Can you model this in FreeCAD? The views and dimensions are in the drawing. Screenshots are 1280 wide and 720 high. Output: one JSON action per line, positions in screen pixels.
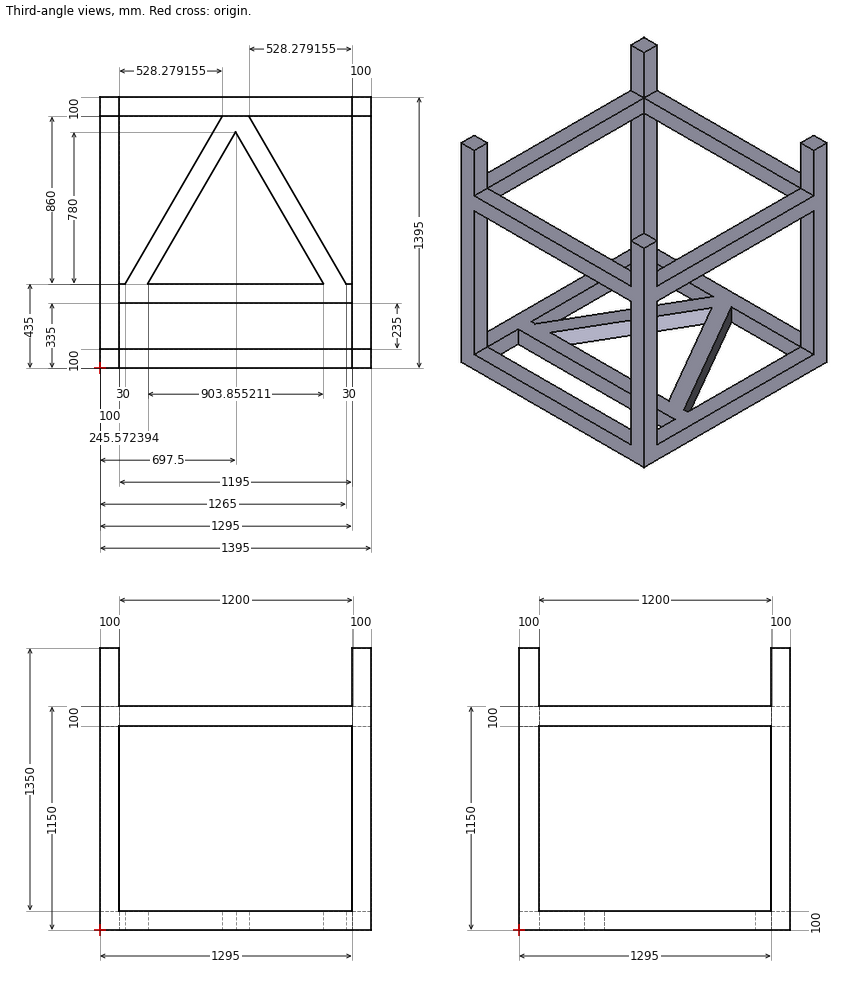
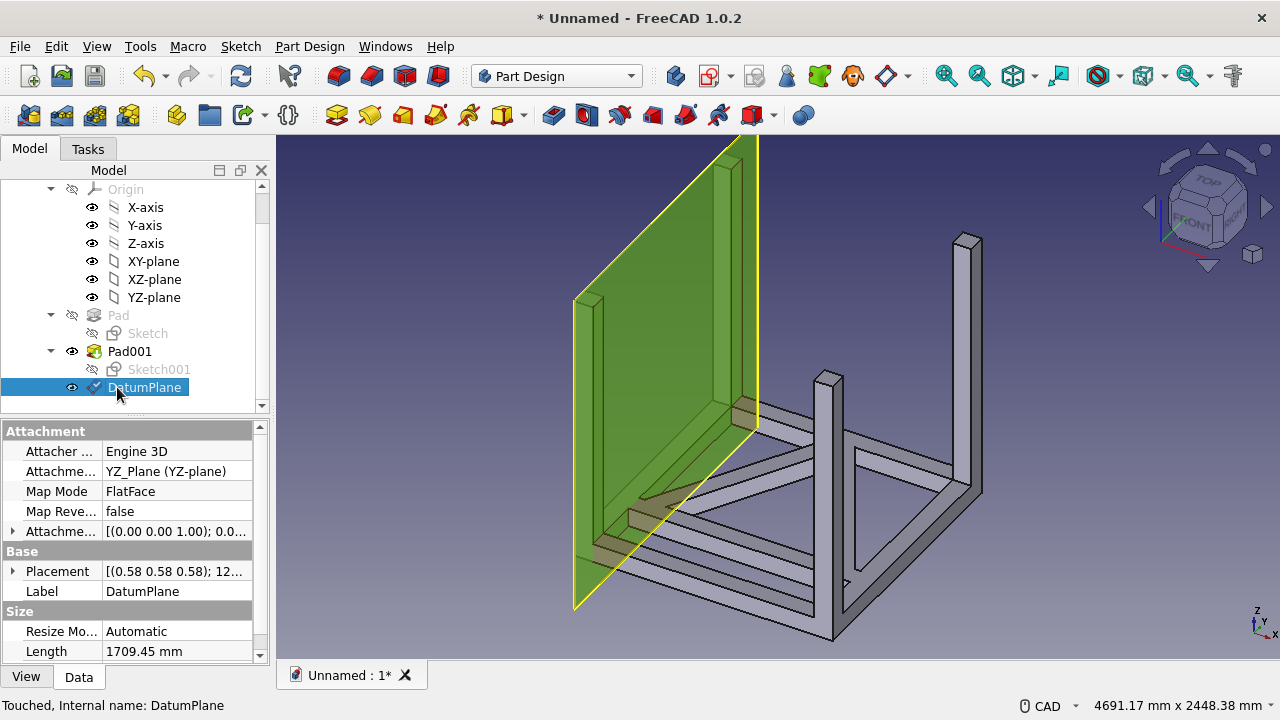
{"action": "left_click", "coordinate": [708, 76]}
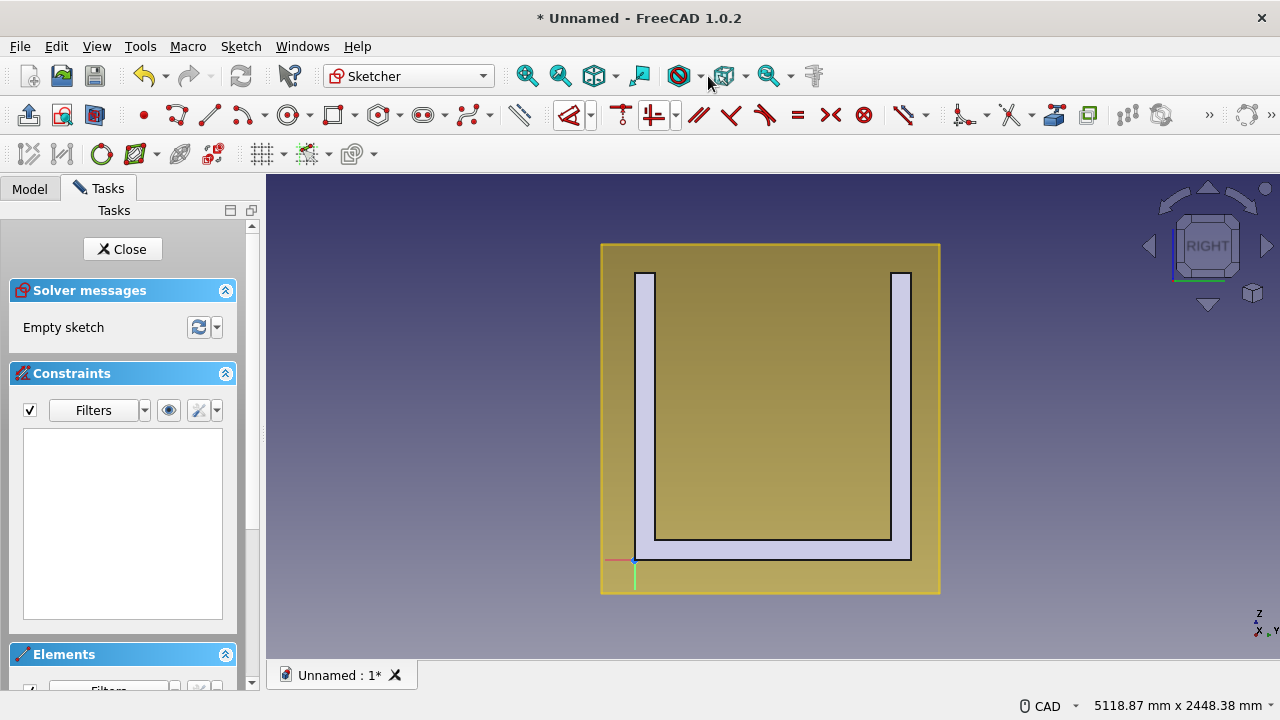
{"action": "left_click", "coordinate": [95, 116]}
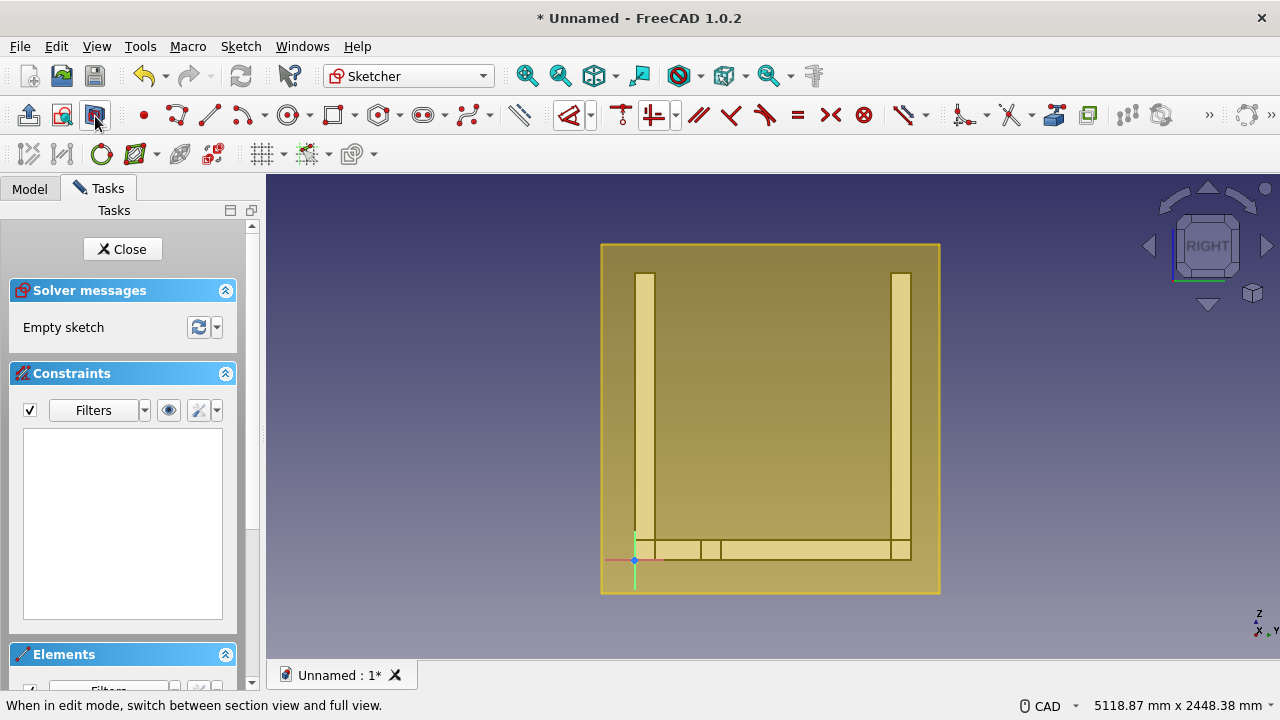
{"action": "left_click", "coordinate": [332, 116]}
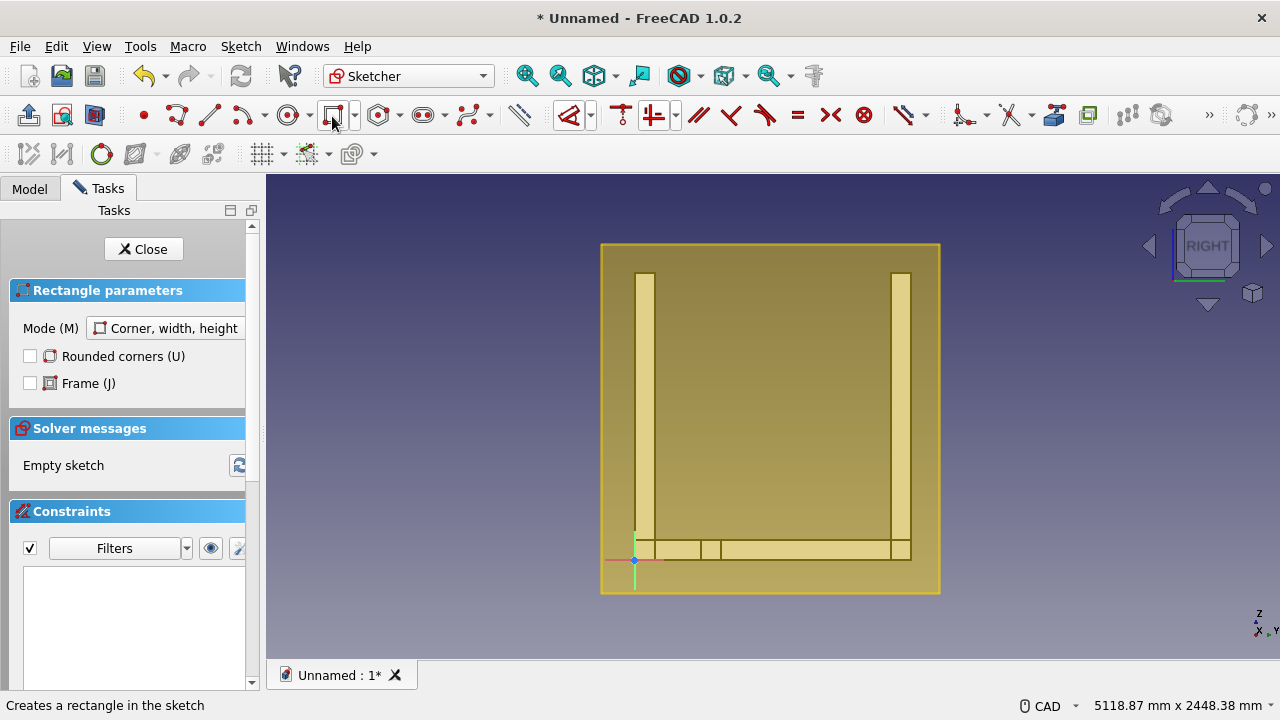
{"action": "left_click", "coordinate": [635, 332]}
{"action": "mouse_move", "coordinate": [655, 352]}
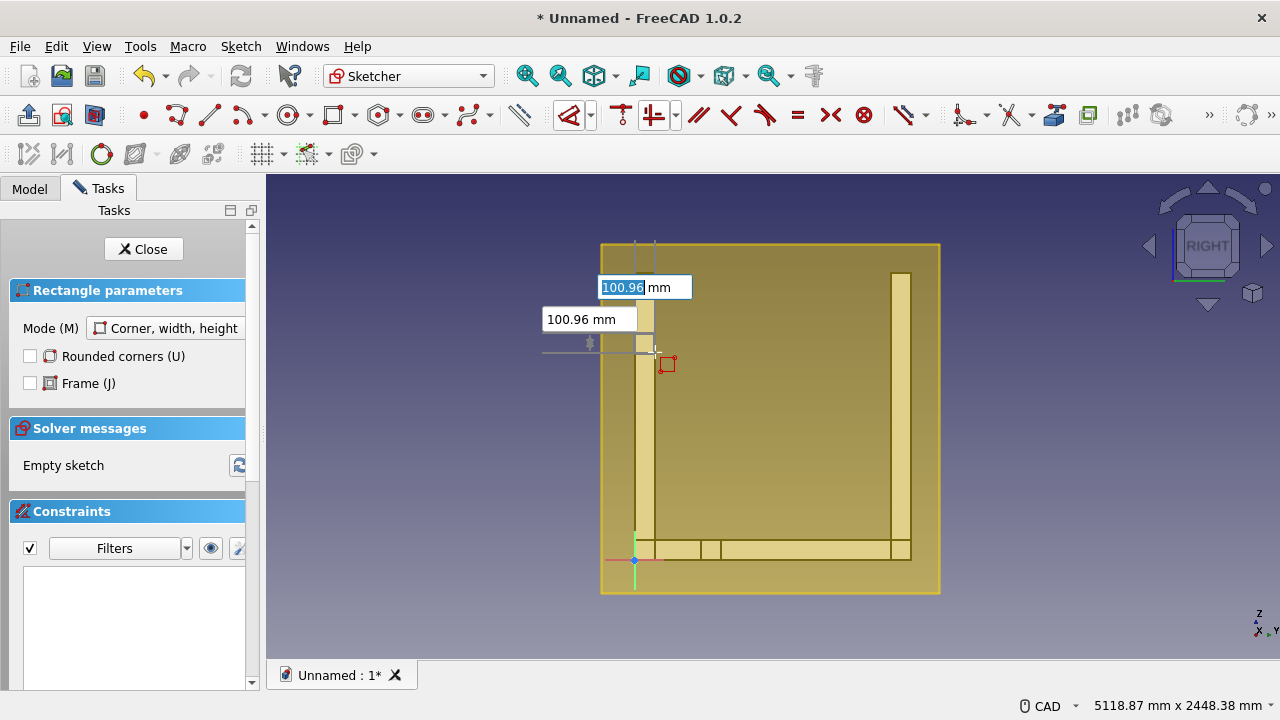
{"action": "type", "text": "100"}
{"action": "key", "text": "Tab"}
{"action": "type", "text": "100"}
{"action": "key", "text": "Return"}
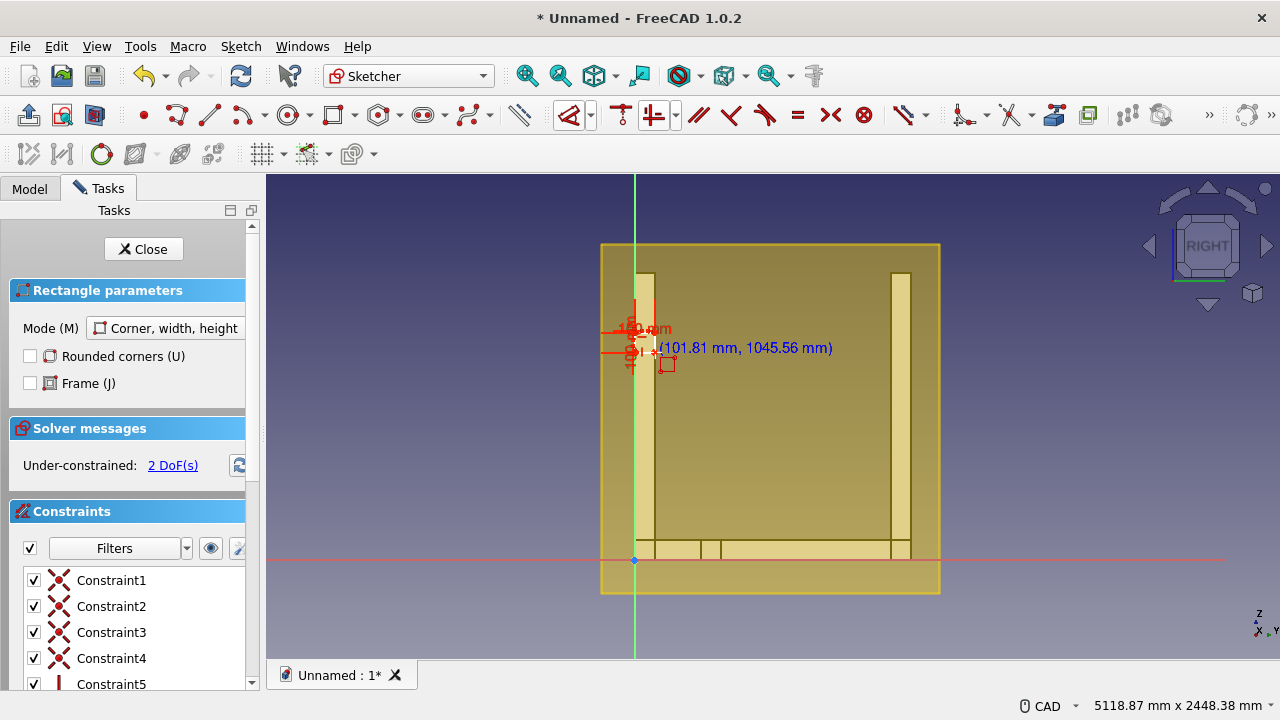
{"action": "left_click", "coordinate": [891, 332]}
{"action": "mouse_move", "coordinate": [911, 352]}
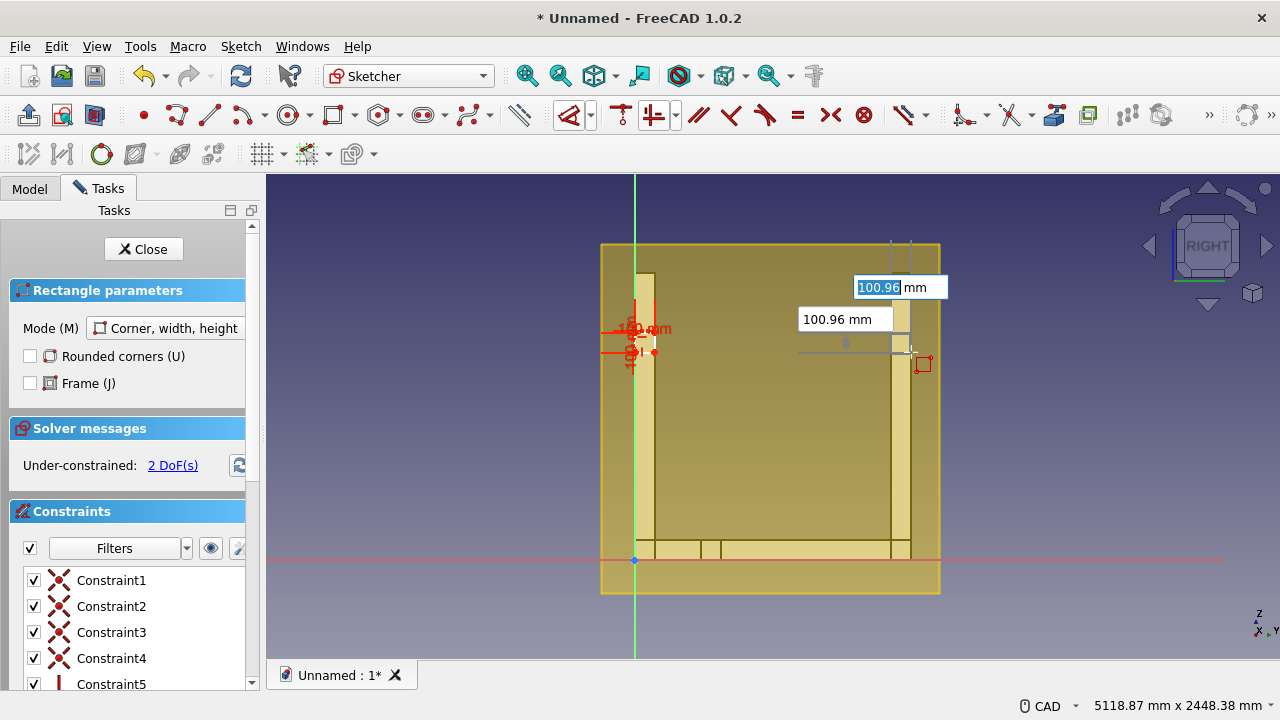
{"action": "type", "text": "100"}
{"action": "key", "text": "Tab"}
{"action": "type", "text": "100"}
{"action": "key", "text": "Return"}
{"action": "key", "text": "Escape"}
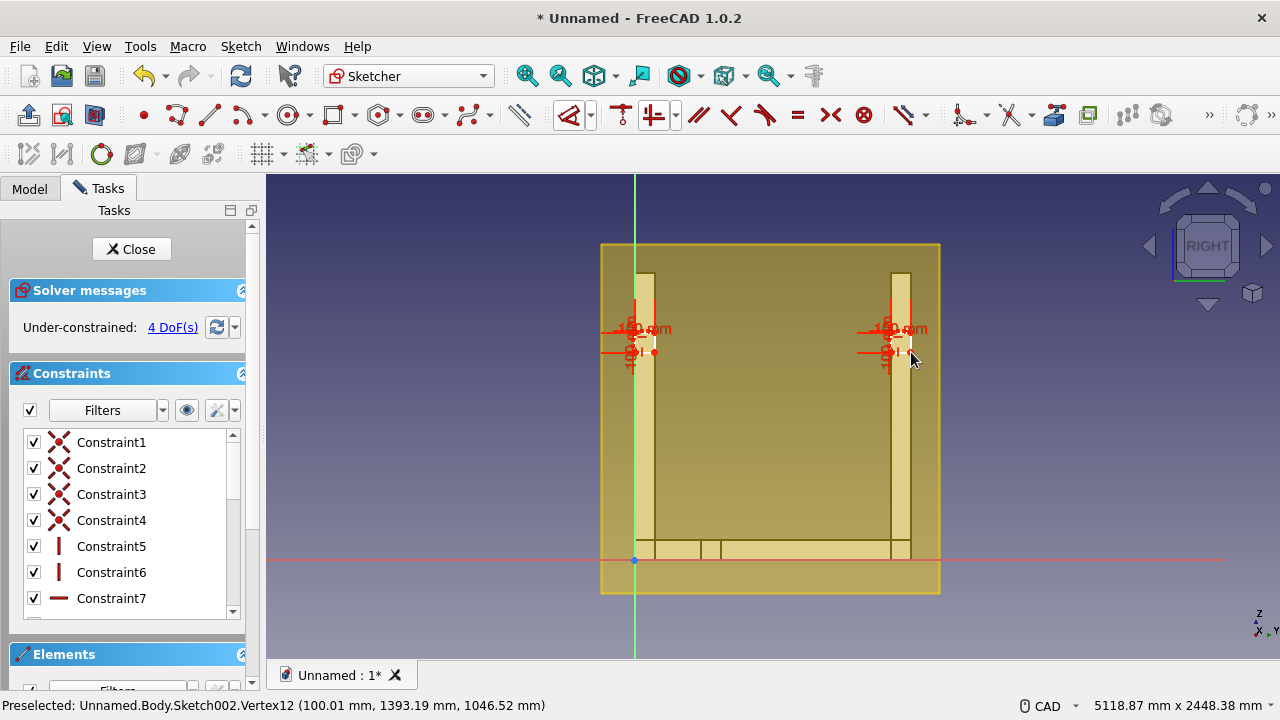
{"action": "left_click", "coordinate": [635, 333]}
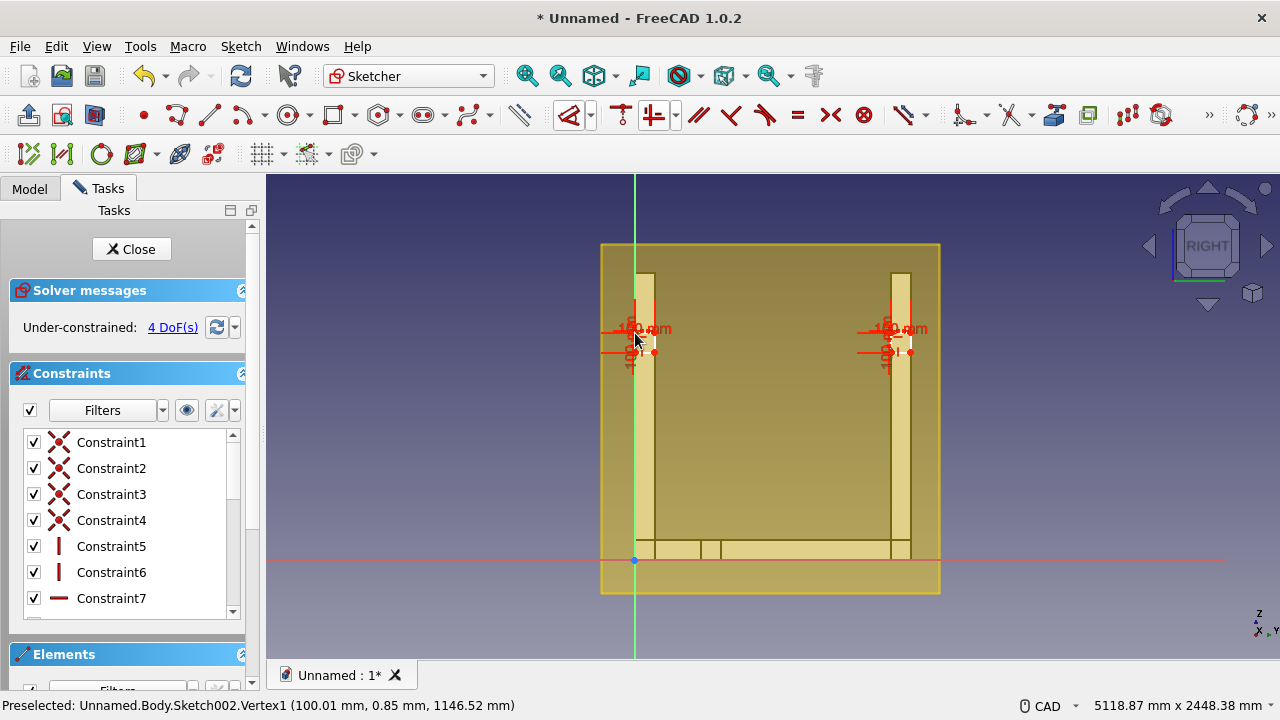
{"action": "left_click", "coordinate": [635, 600]}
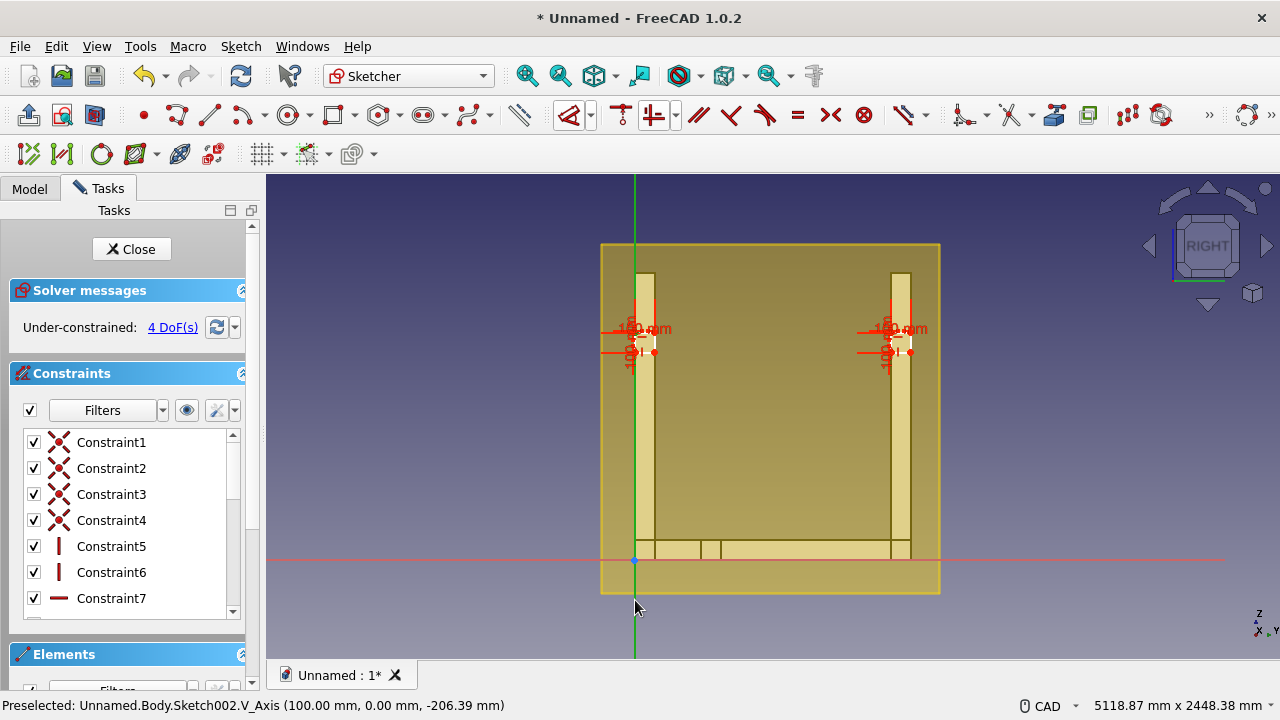
{"action": "left_click", "coordinate": [621, 116]}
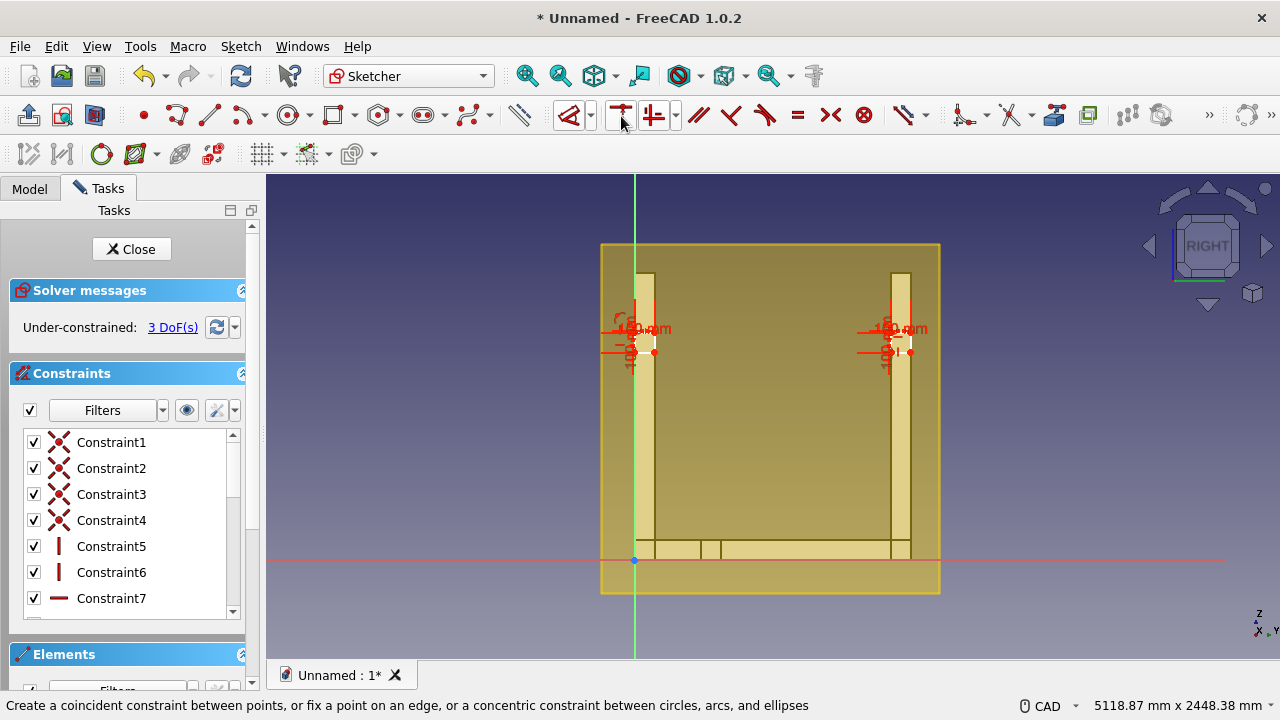
{"action": "left_click", "coordinate": [635, 333]}